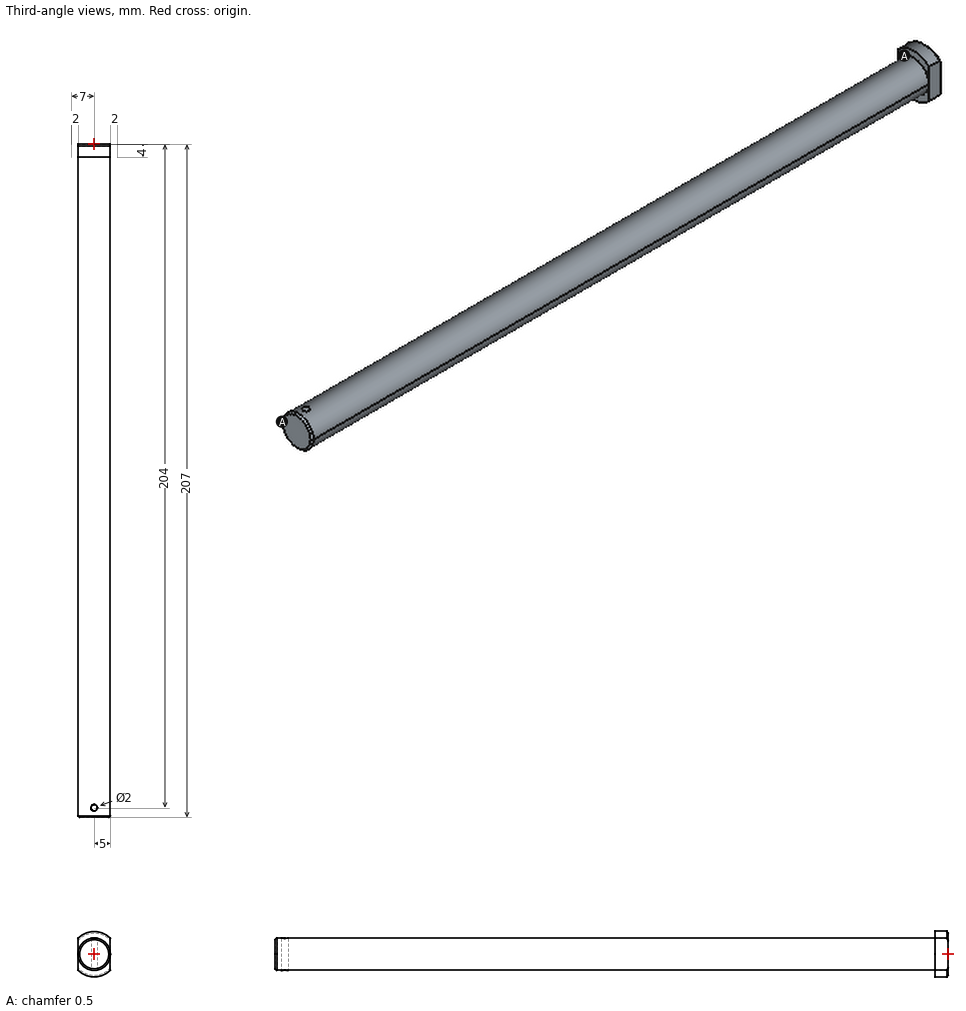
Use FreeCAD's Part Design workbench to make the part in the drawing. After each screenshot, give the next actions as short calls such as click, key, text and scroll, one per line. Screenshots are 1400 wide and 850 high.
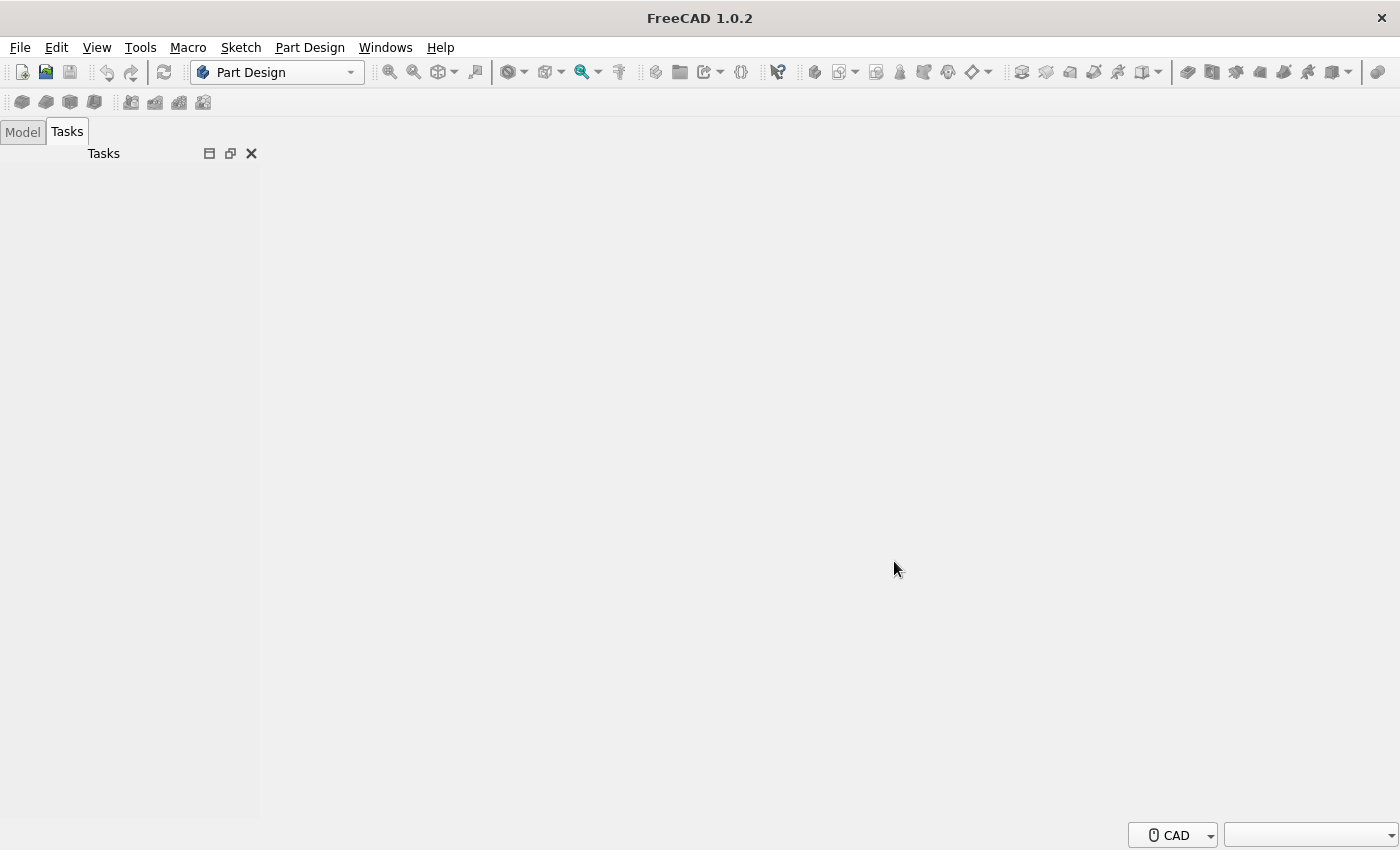
click(22, 72)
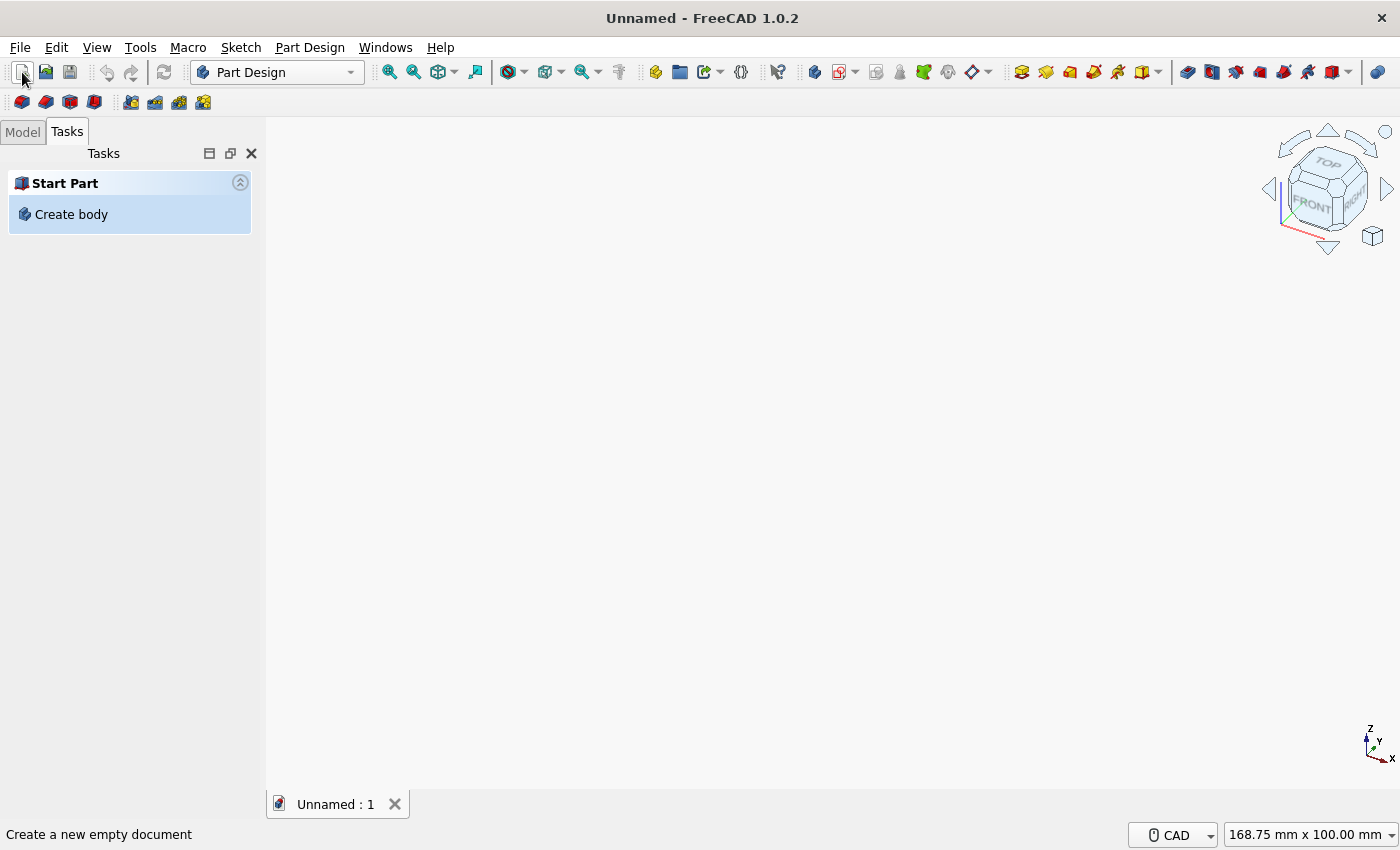
click(840, 72)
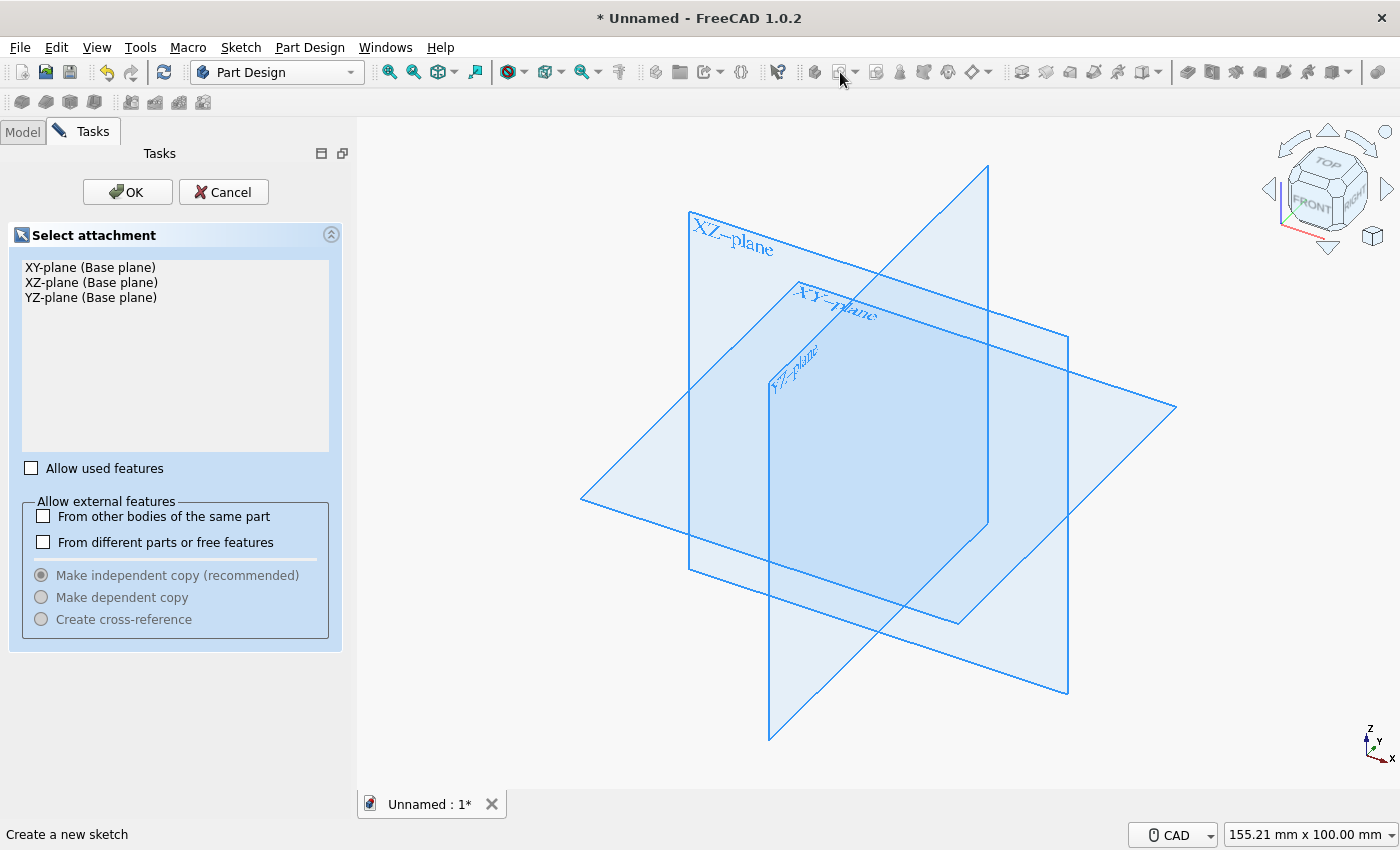
click(82, 268)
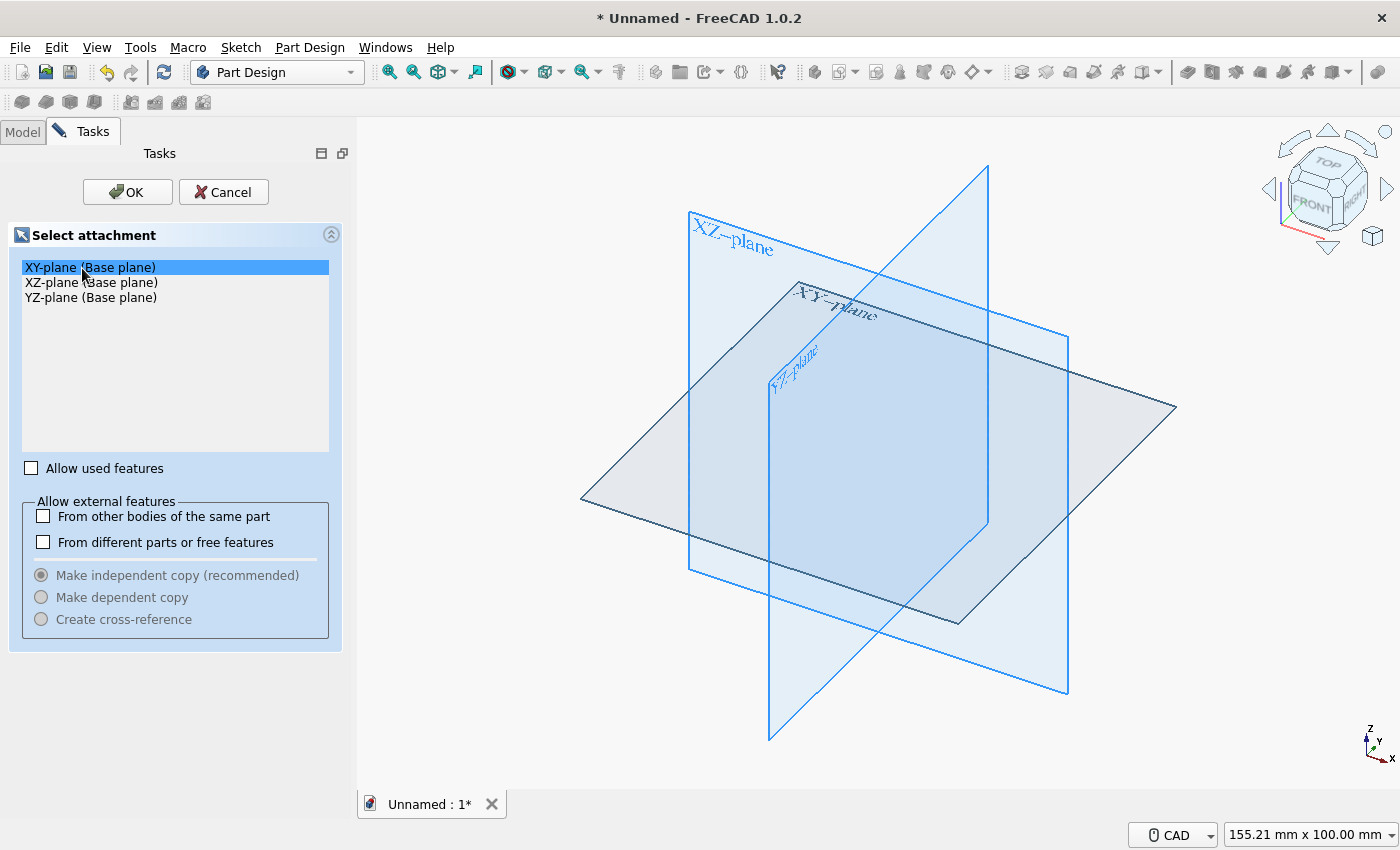
click(128, 192)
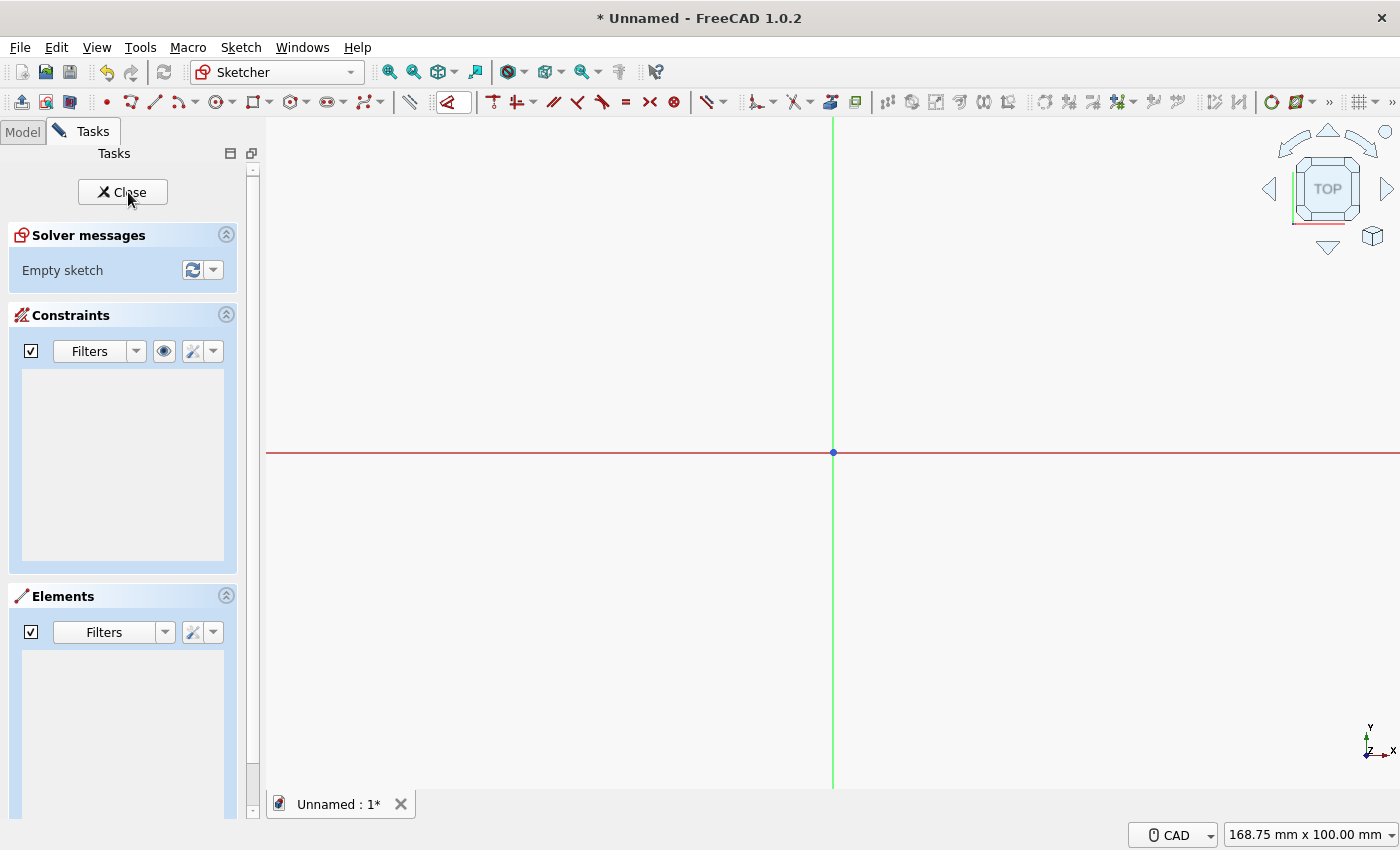
scroll(725, 153, down, 6)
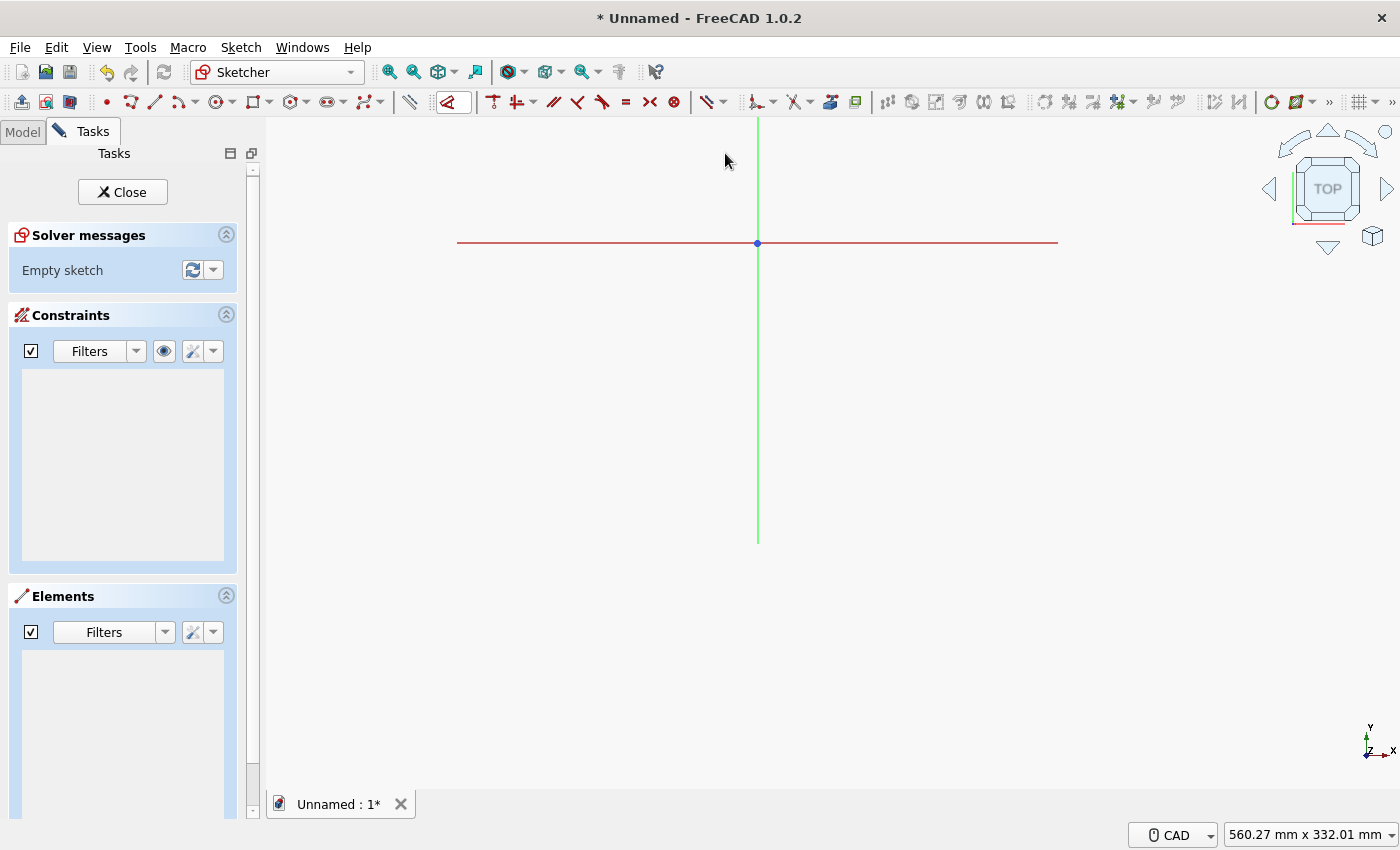
click(132, 102)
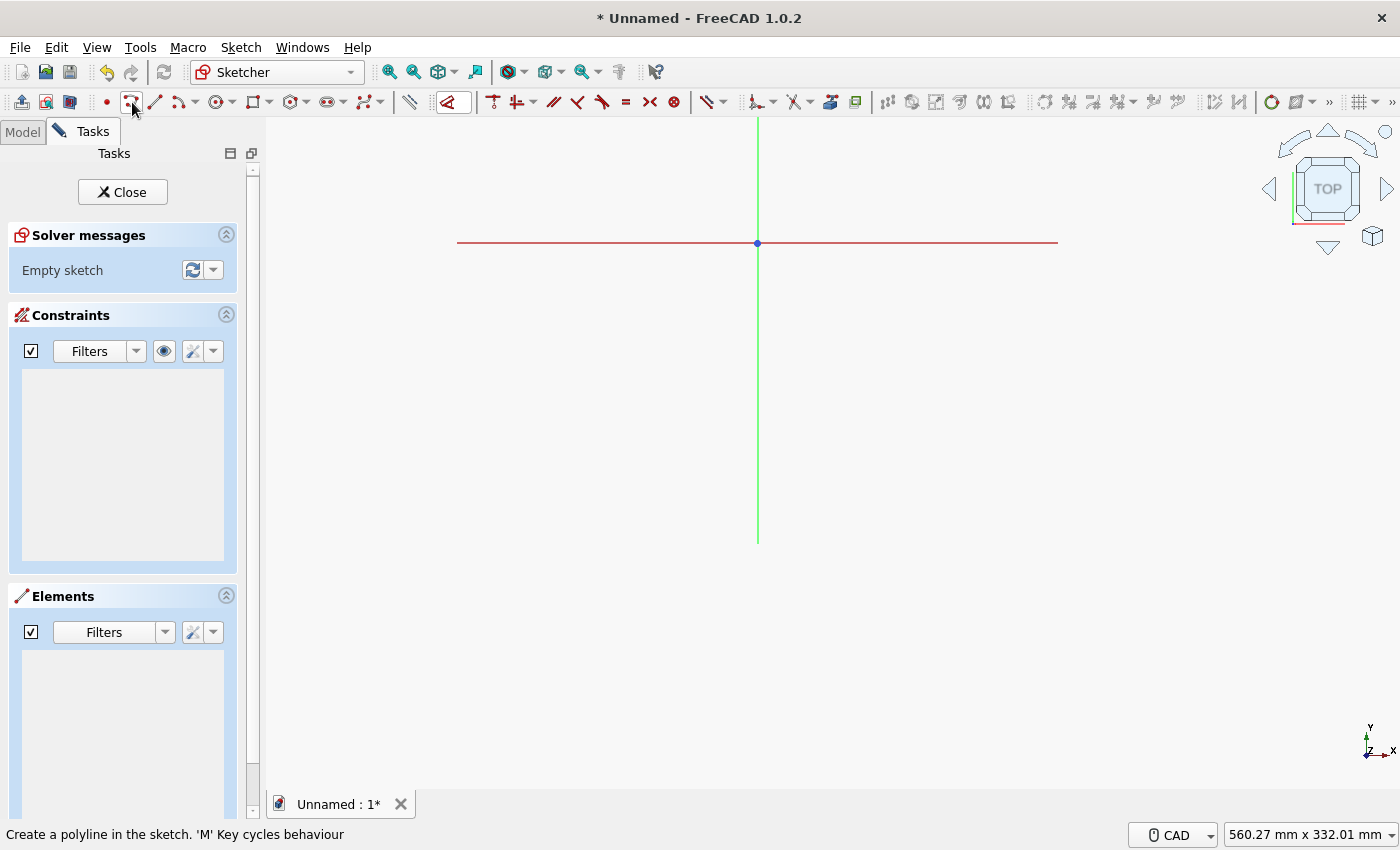
click(758, 243)
click(767, 662)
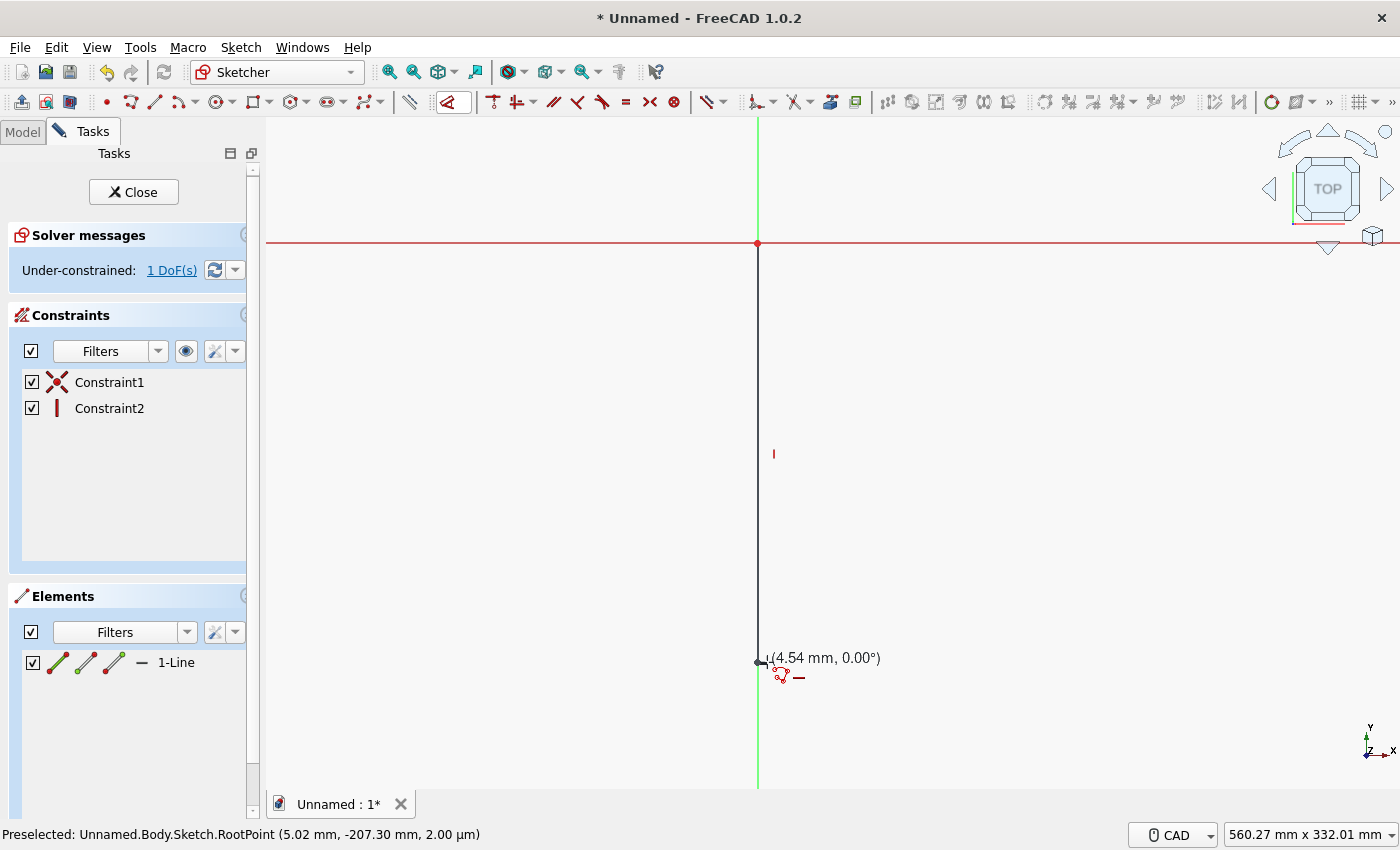
scroll(768, 662, up, 3)